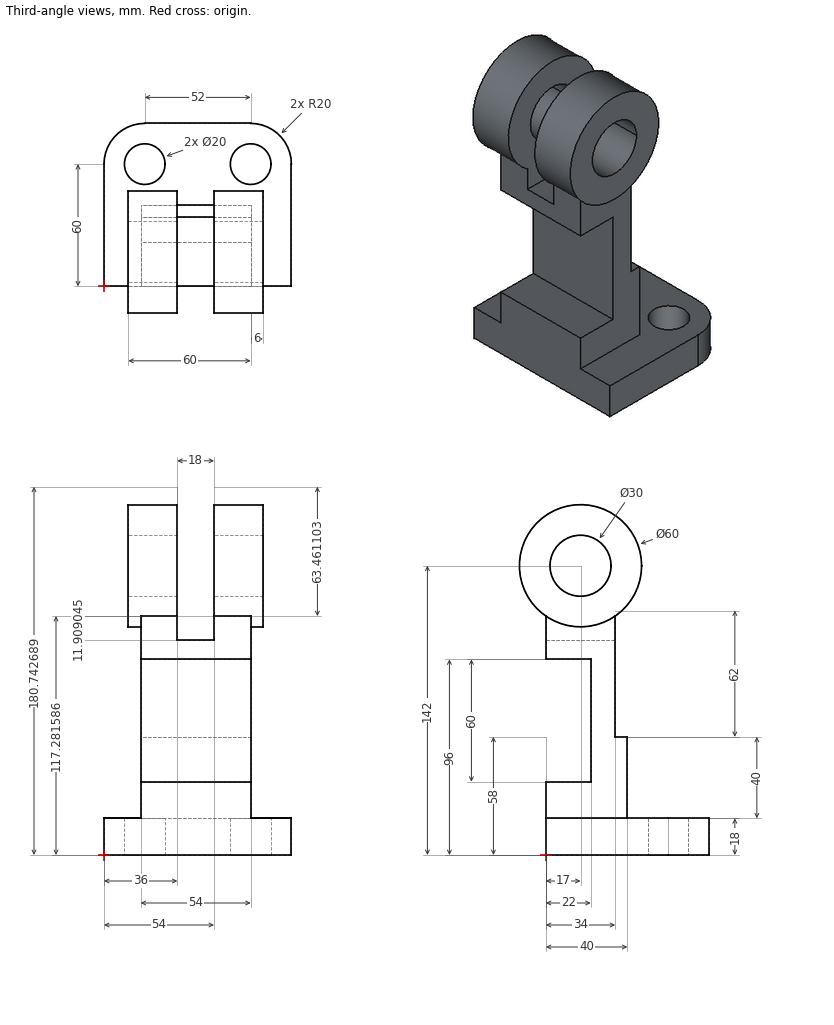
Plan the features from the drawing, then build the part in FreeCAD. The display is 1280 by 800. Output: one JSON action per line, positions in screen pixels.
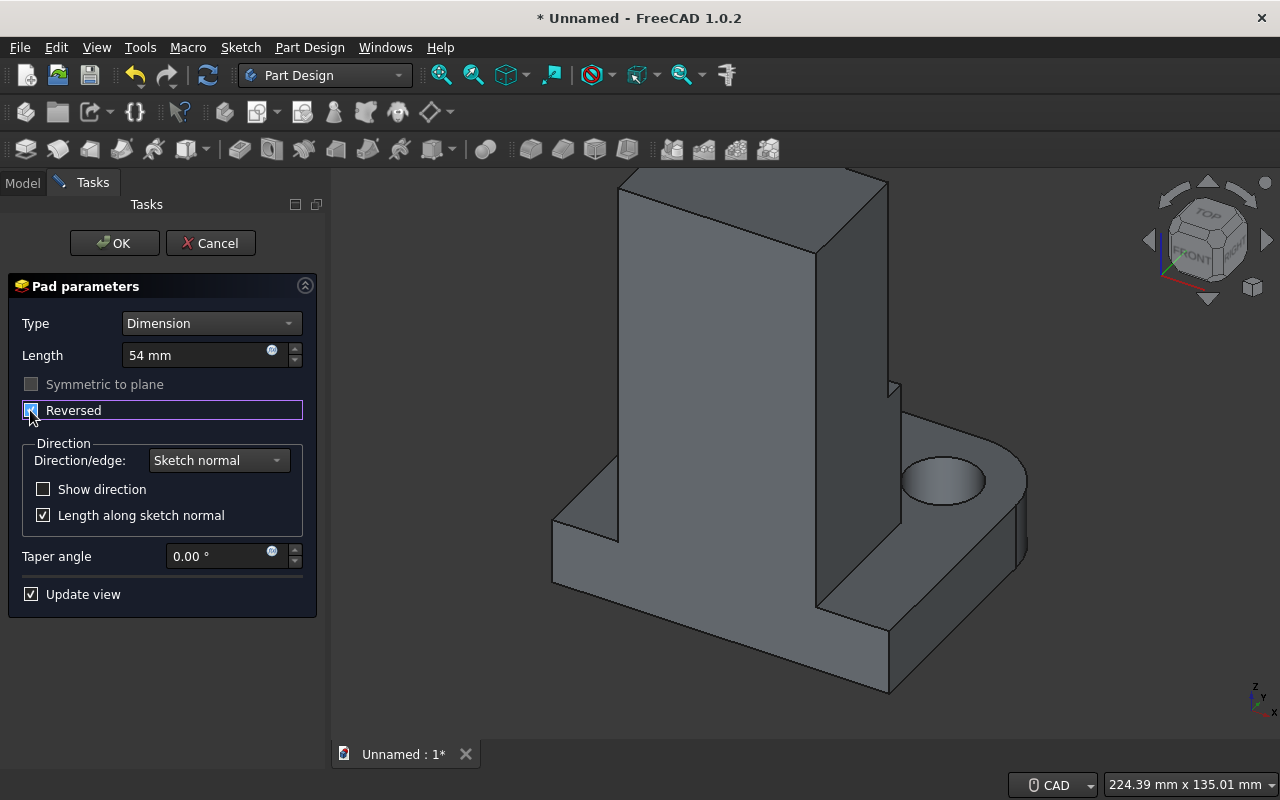
{"action": "left_click", "coordinate": [115, 243]}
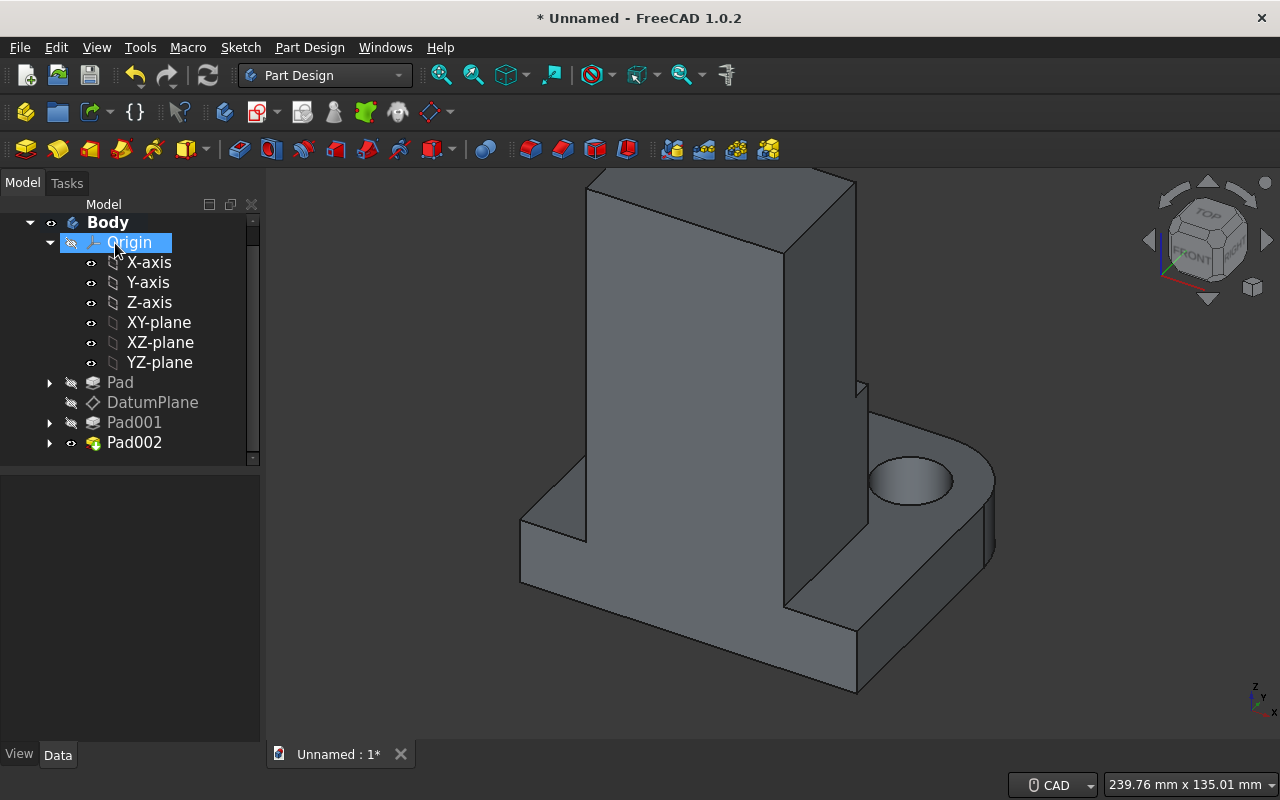
{"action": "left_click", "coordinate": [442, 76]}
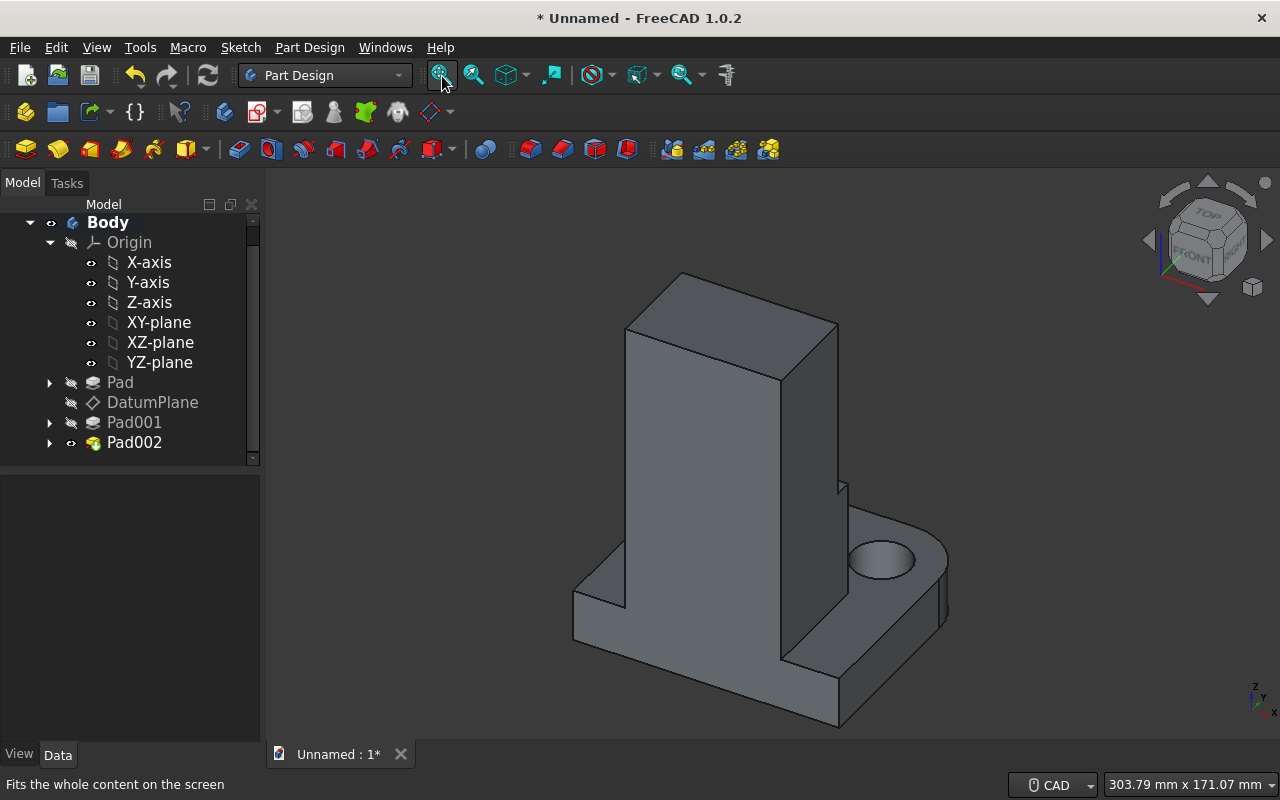
{"action": "left_click", "coordinate": [815, 566]}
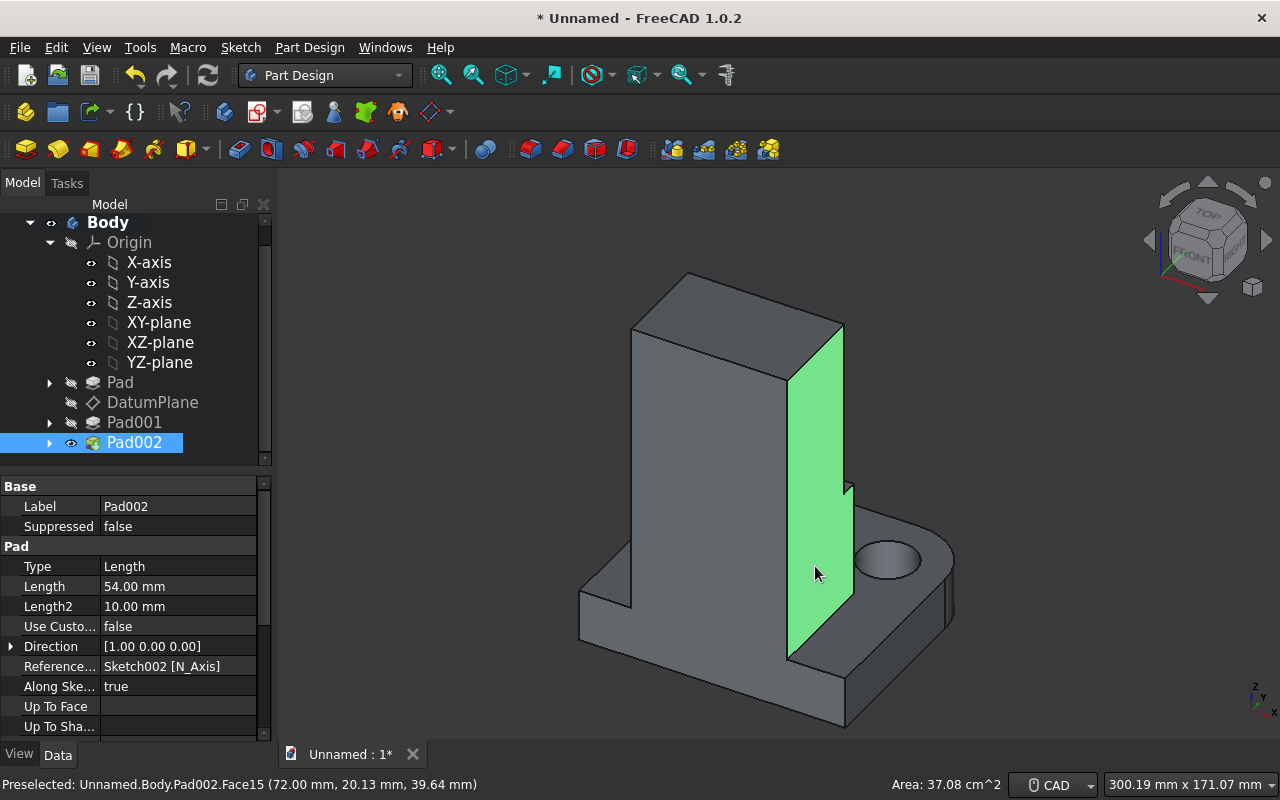
{"action": "left_click", "coordinate": [258, 112]}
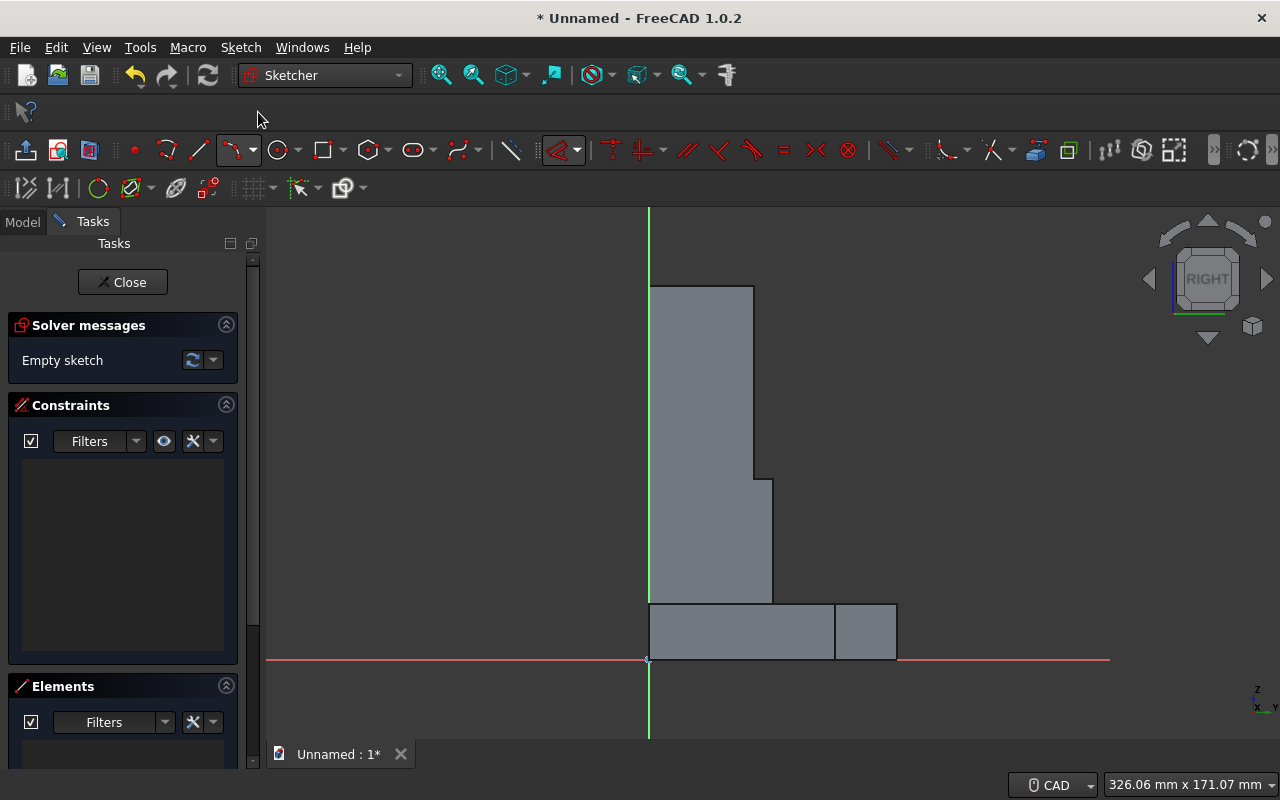
{"action": "left_click", "coordinate": [90, 150]}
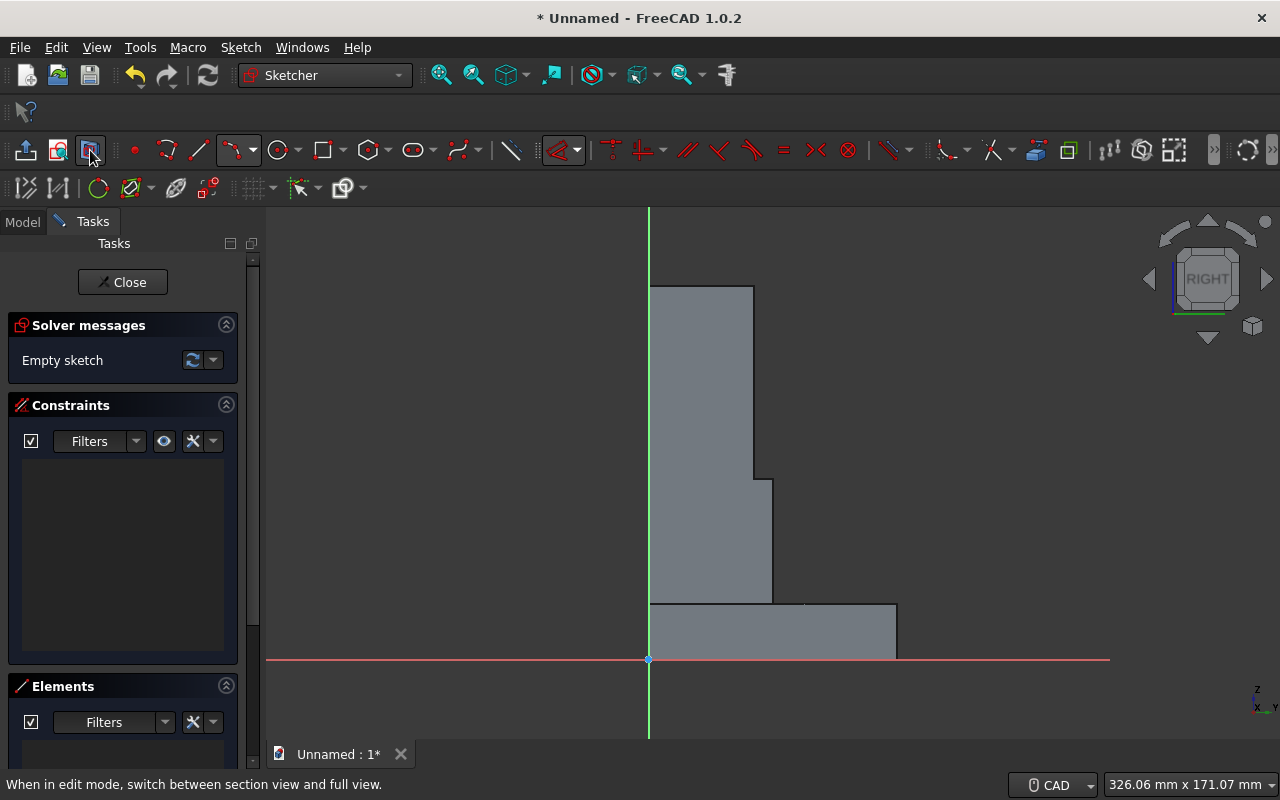
{"action": "left_click", "coordinate": [324, 150]}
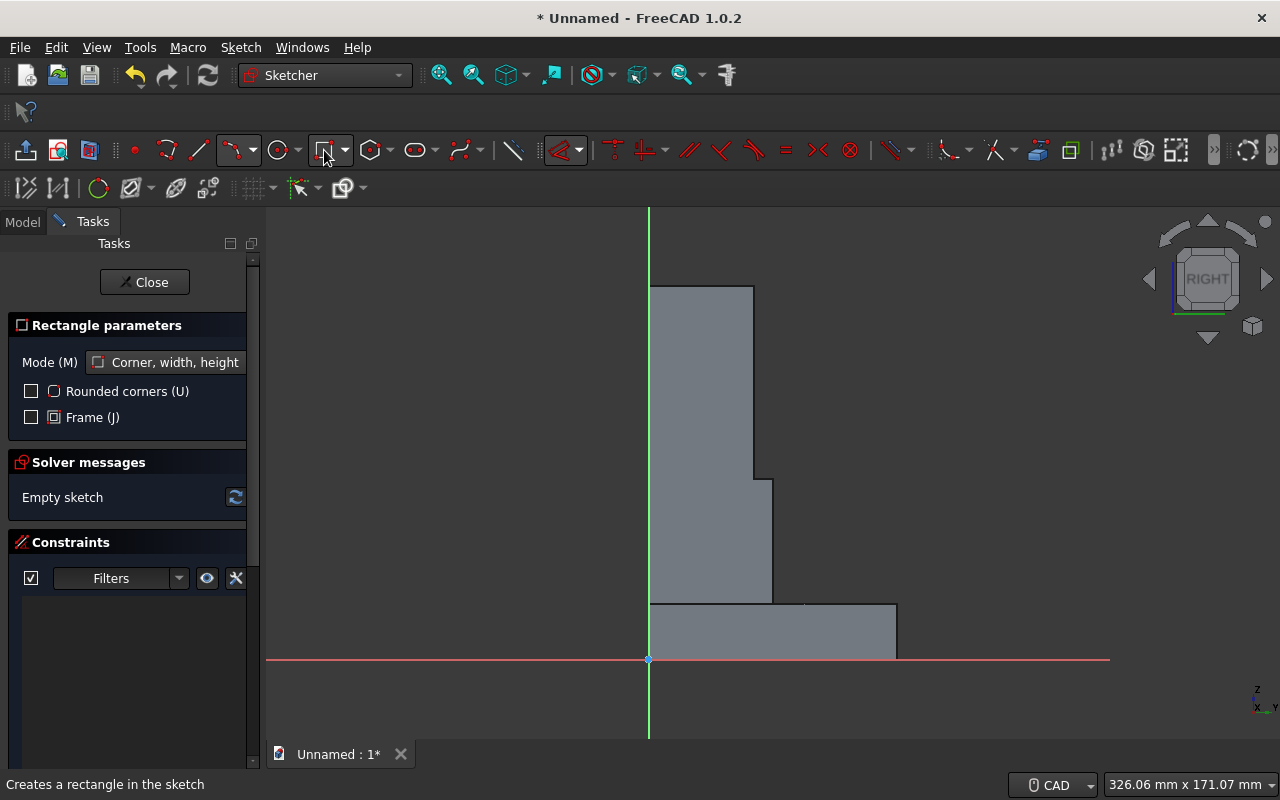
{"action": "left_click", "coordinate": [649, 361]}
{"action": "mouse_move", "coordinate": [717, 548]}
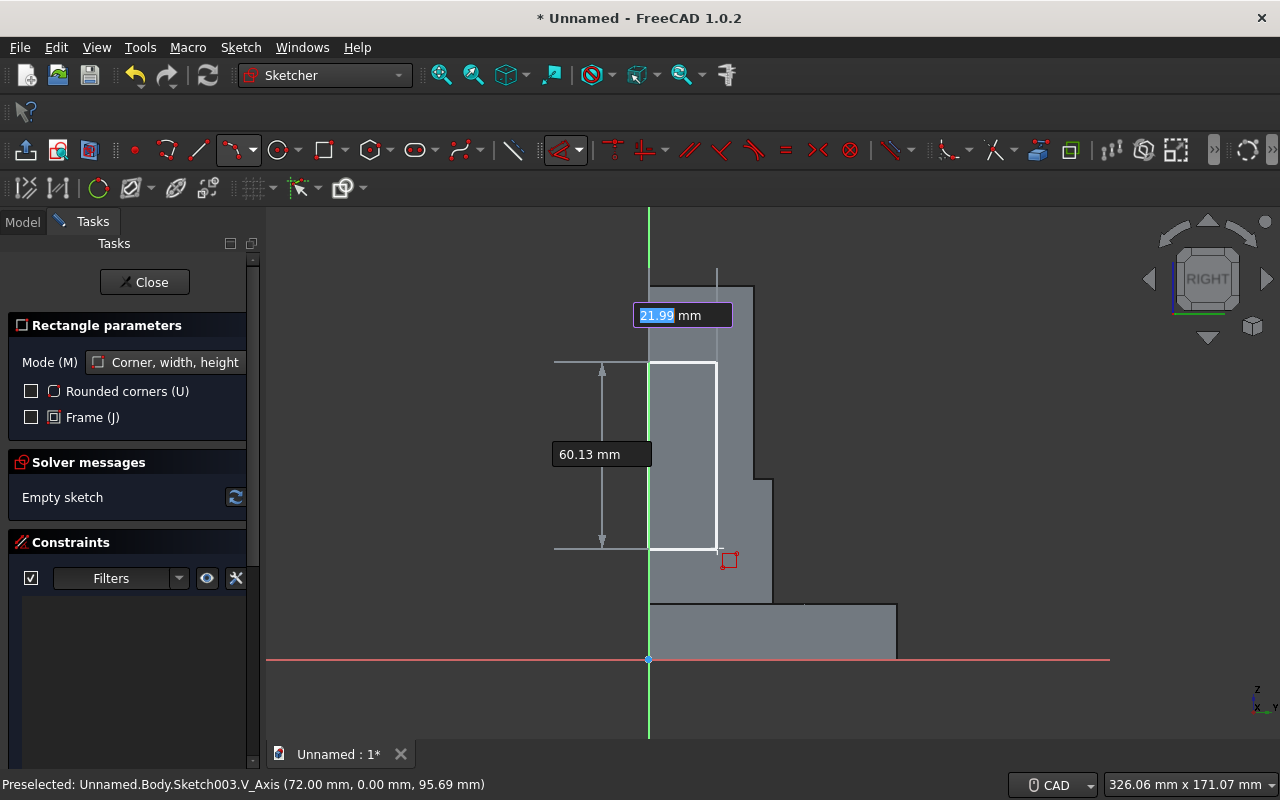
{"action": "type", "text": "22"}
{"action": "key", "text": "Tab"}
{"action": "type", "text": "60"}
{"action": "key", "text": "Return"}
{"action": "key", "text": "Escape"}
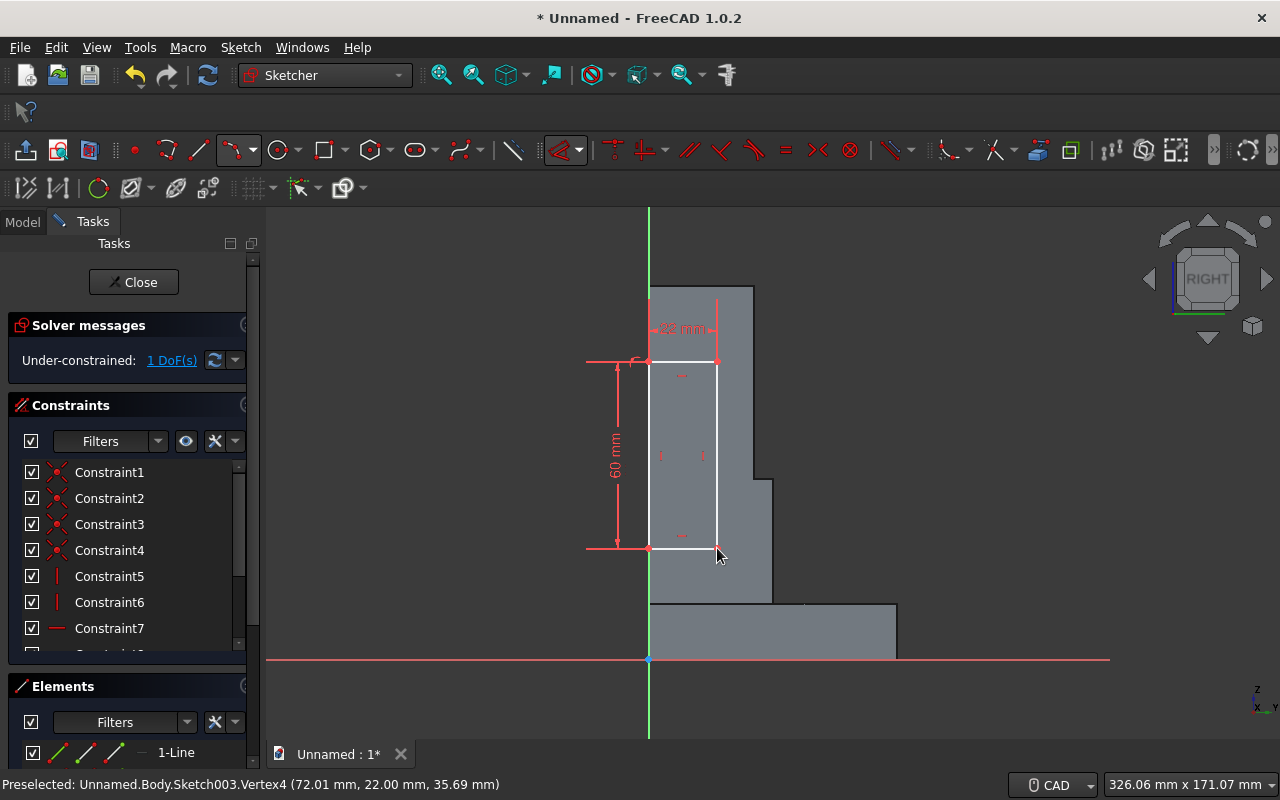
{"action": "left_click", "coordinate": [649, 362]}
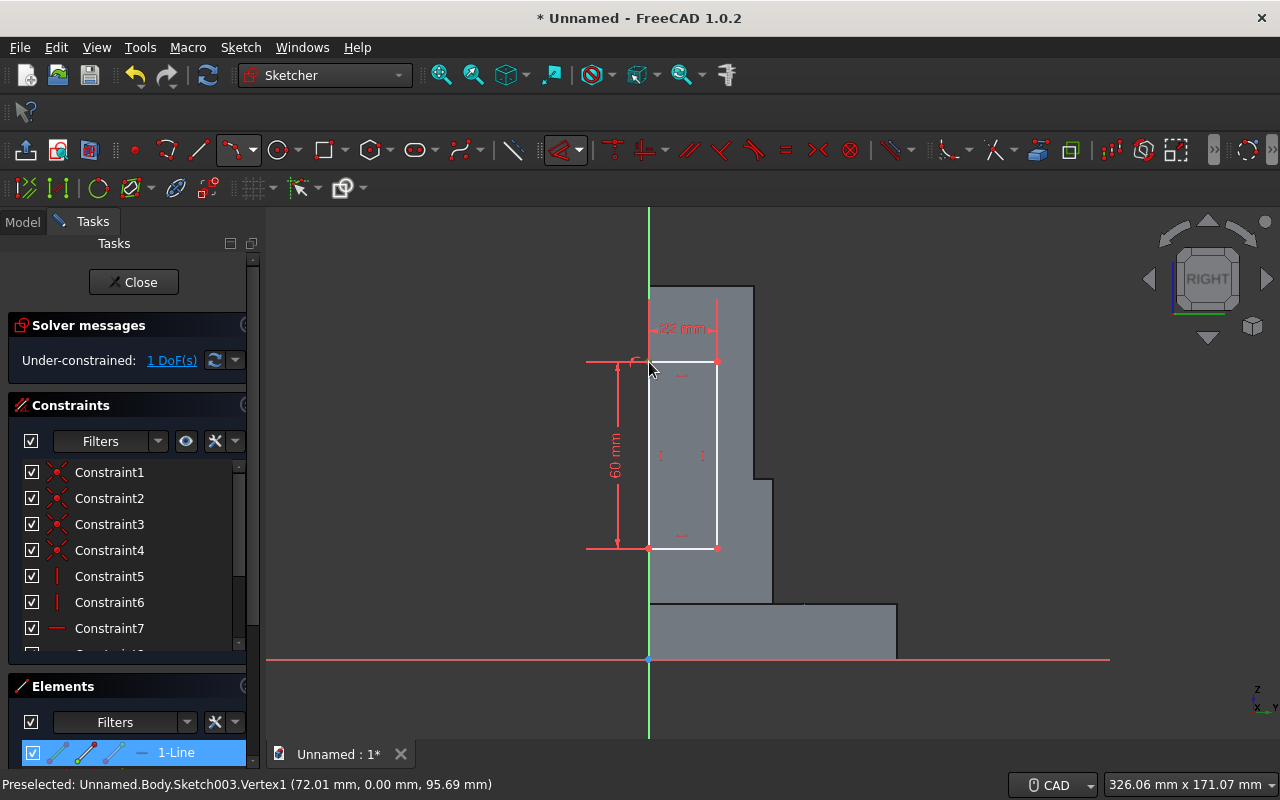
{"action": "key", "text": "i"}